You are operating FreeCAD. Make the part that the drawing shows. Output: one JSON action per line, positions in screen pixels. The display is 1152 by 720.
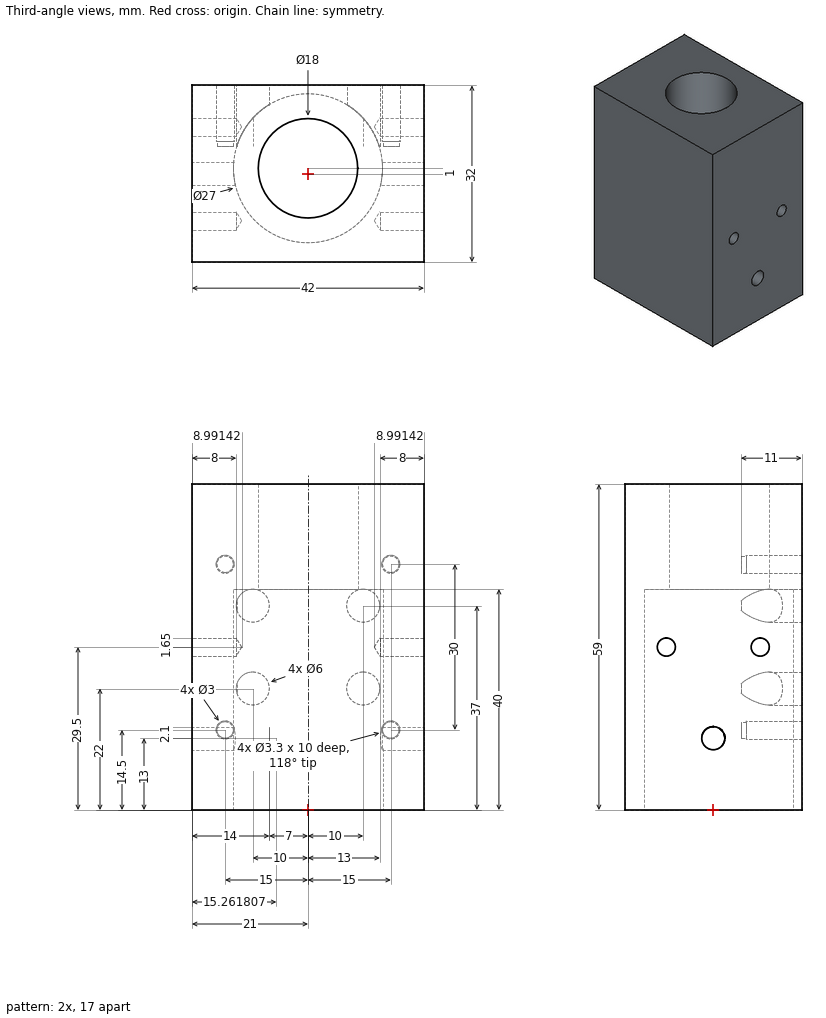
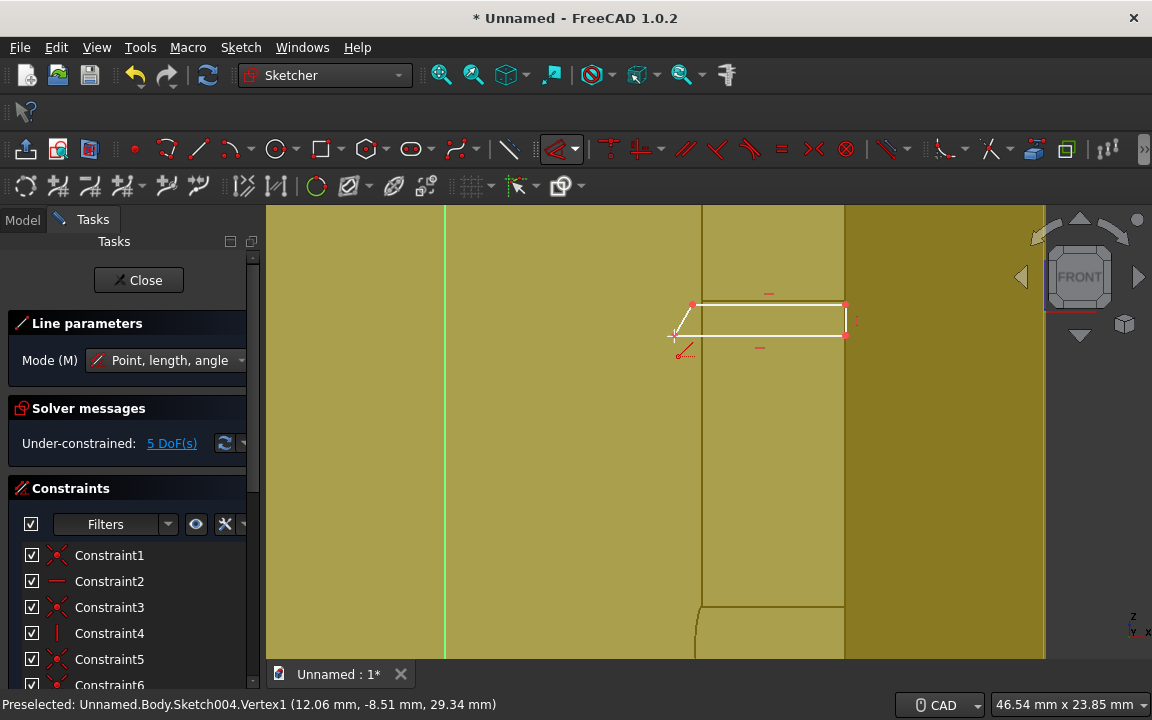
{"action": "left_click", "coordinate": [862, 333]}
{"action": "left_click", "coordinate": [913, 333]}
{"action": "key", "text": "Escape"}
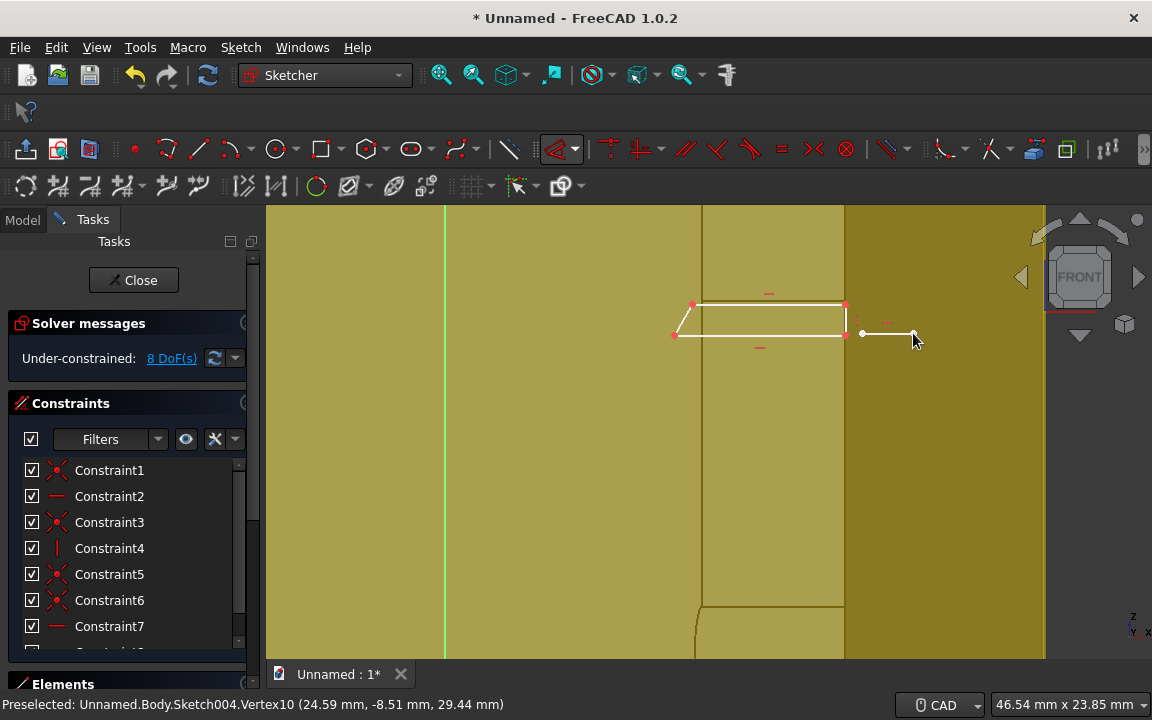
{"action": "left_click", "coordinate": [877, 334]}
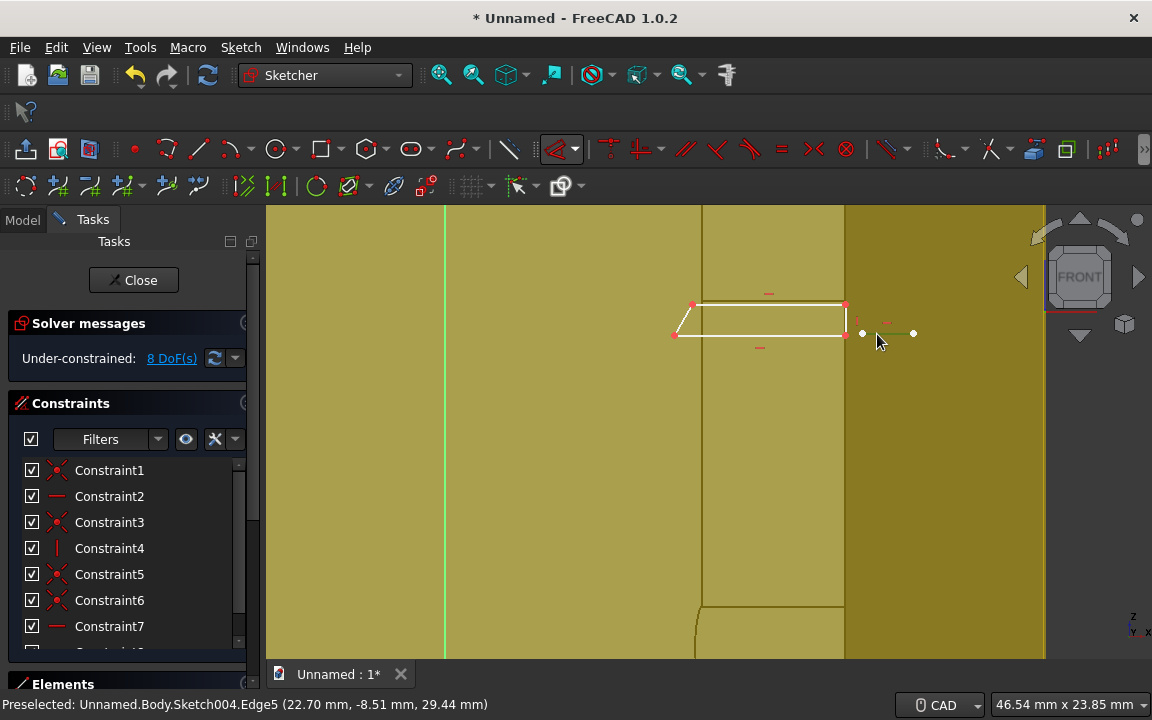
{"action": "left_click", "coordinate": [510, 150]}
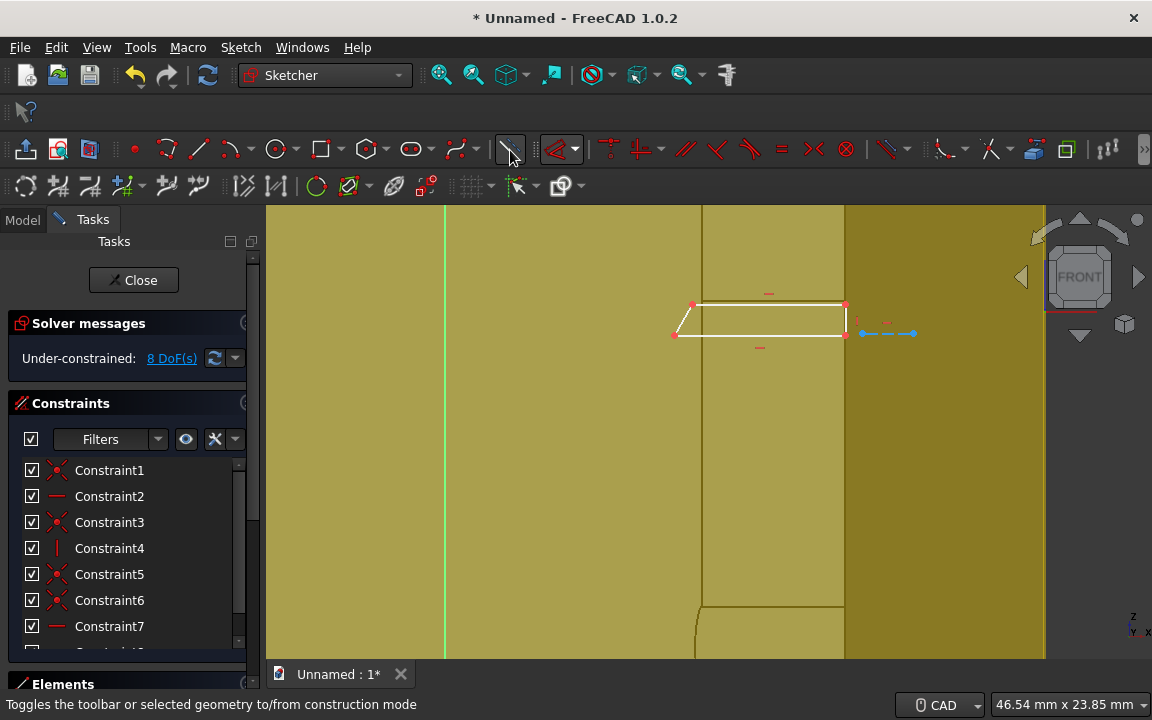
{"action": "left_click", "coordinate": [738, 305]}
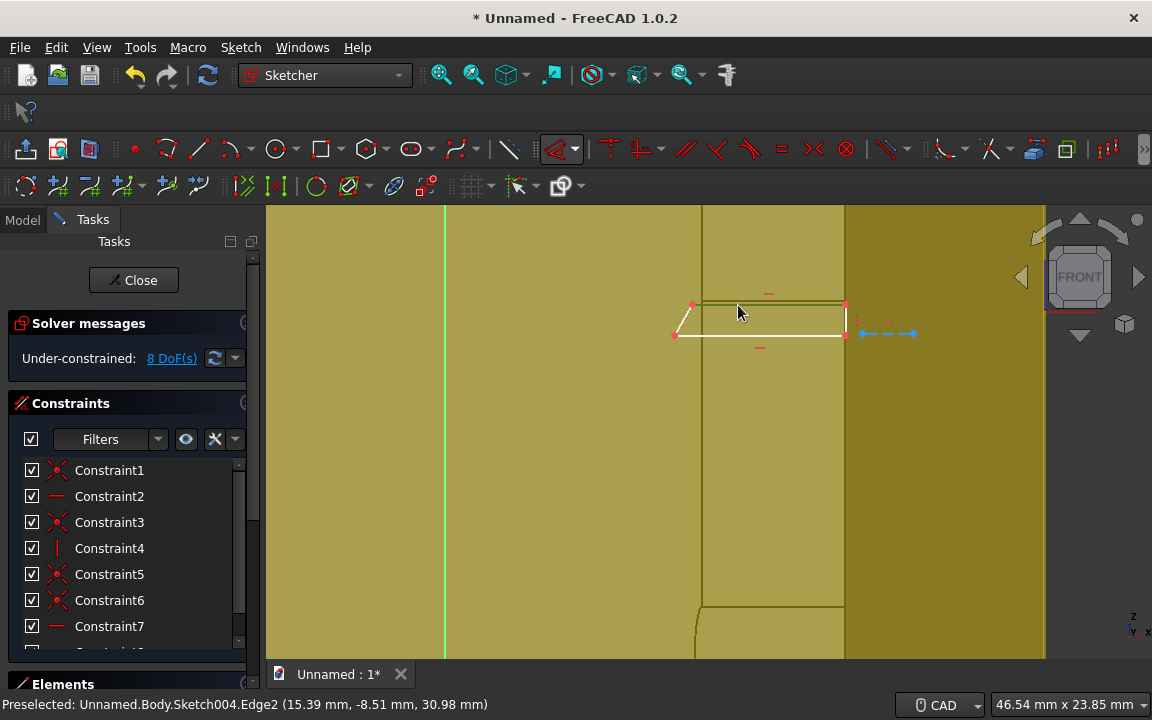
{"action": "left_click", "coordinate": [578, 150]}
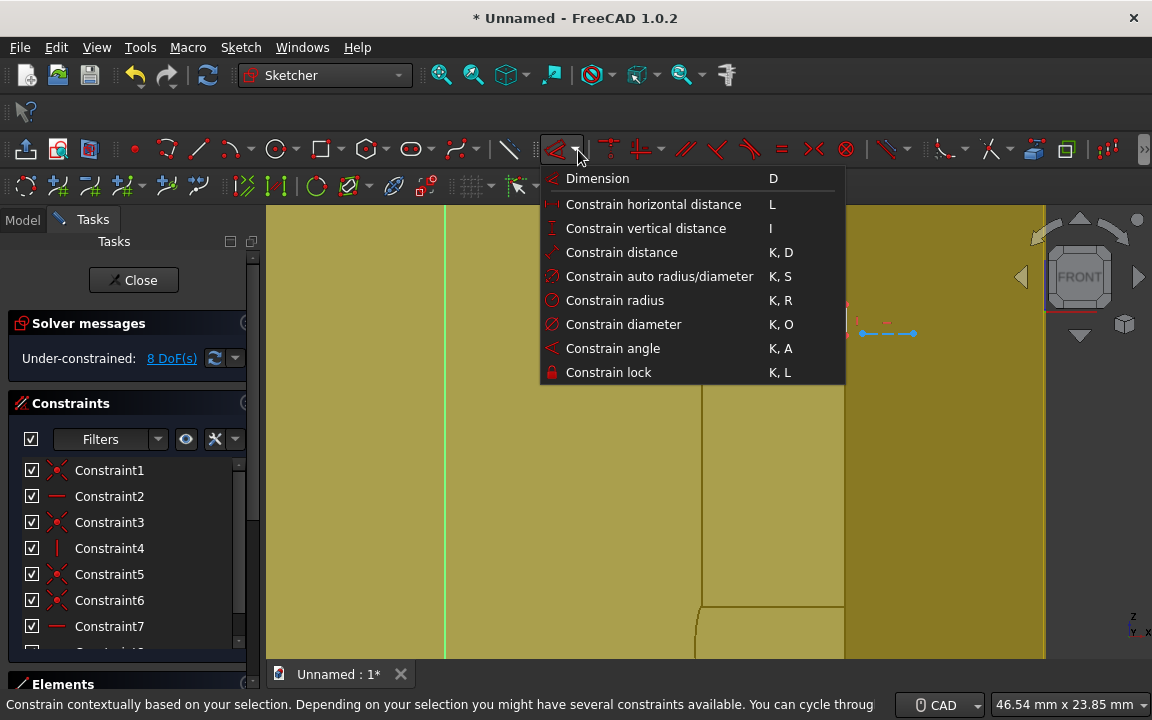
{"action": "left_click", "coordinate": [693, 204]}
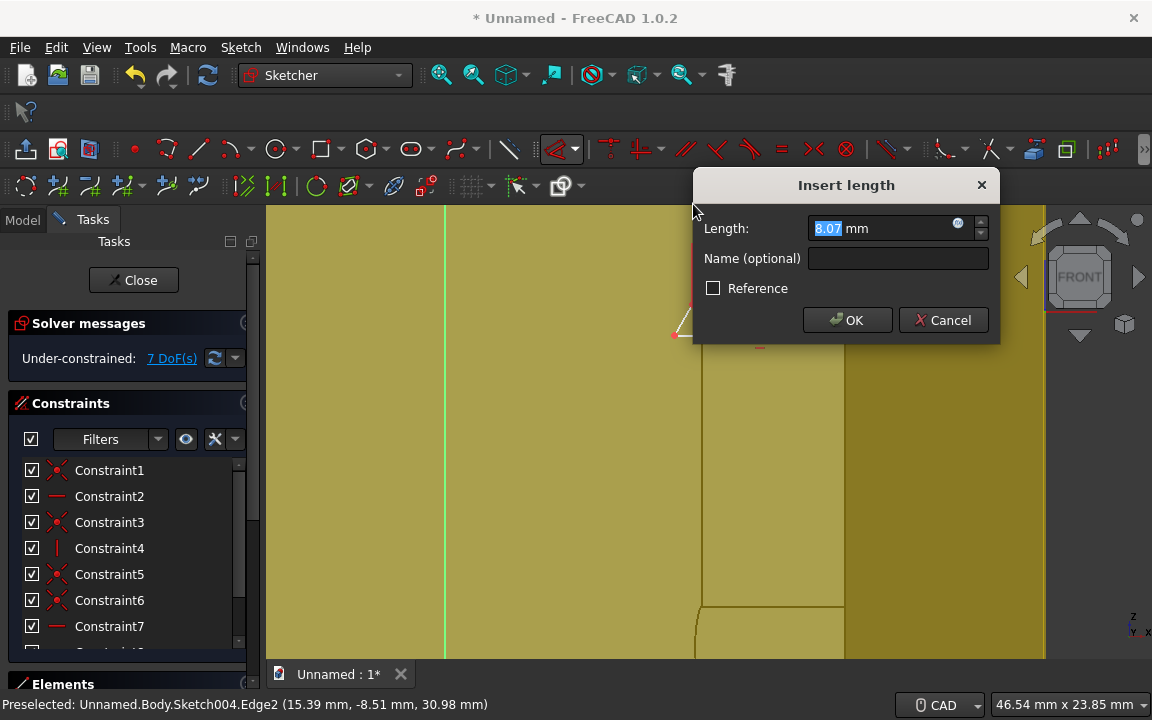
{"action": "type", "text": "8"}
{"action": "key", "text": "Return"}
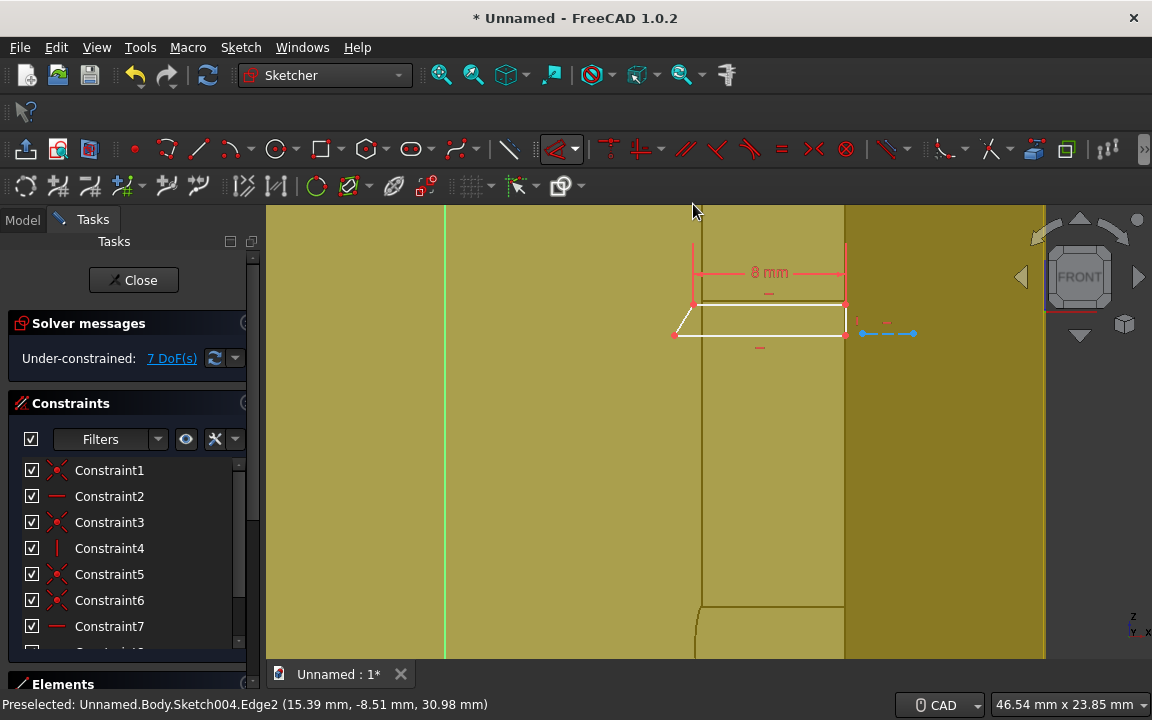
{"action": "left_click", "coordinate": [694, 305]}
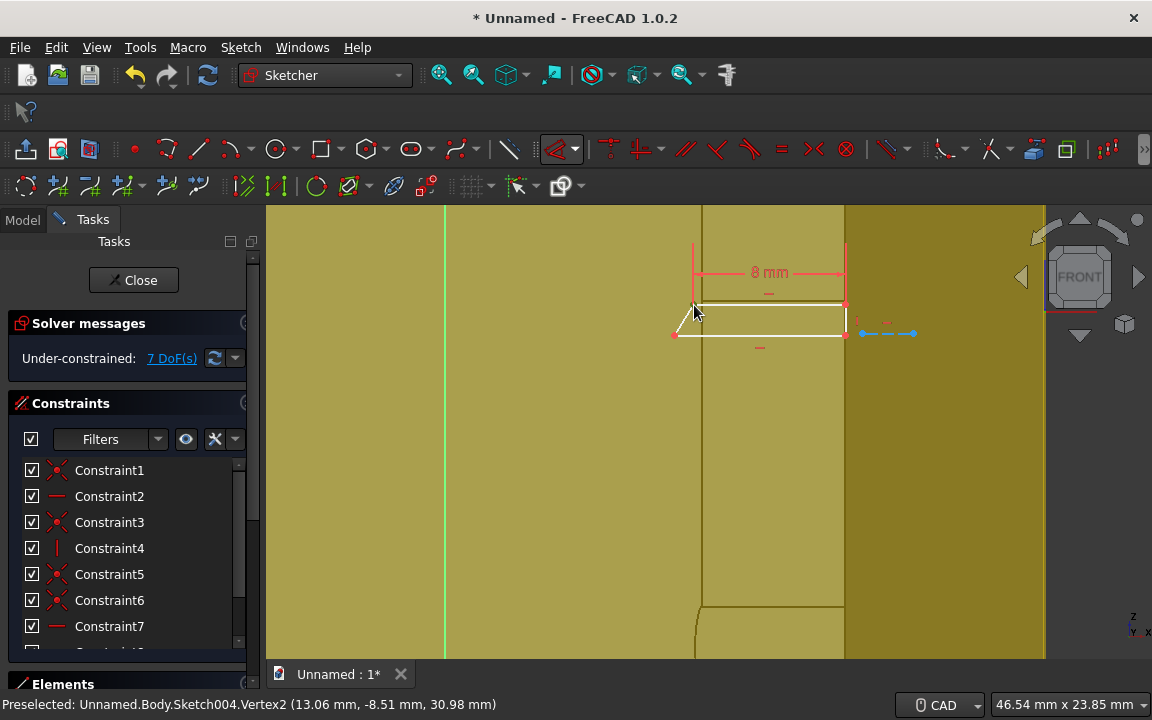
{"action": "key", "text": "l"}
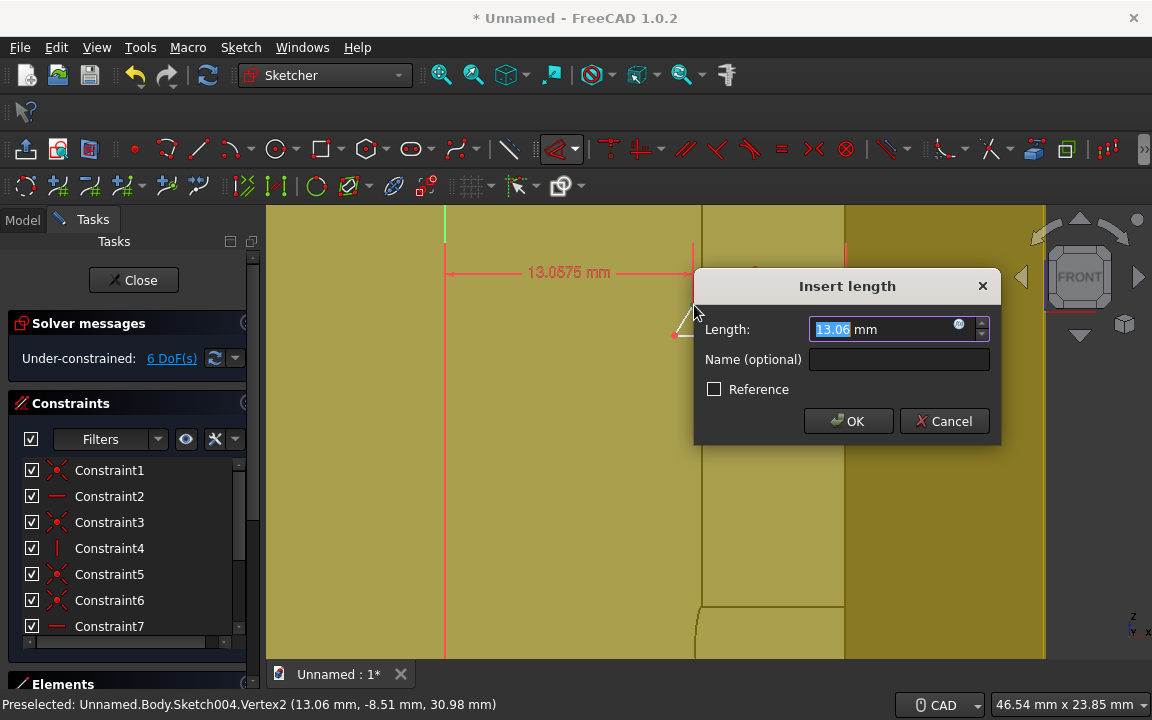
{"action": "type", "text": "13"}
{"action": "key", "text": "Return"}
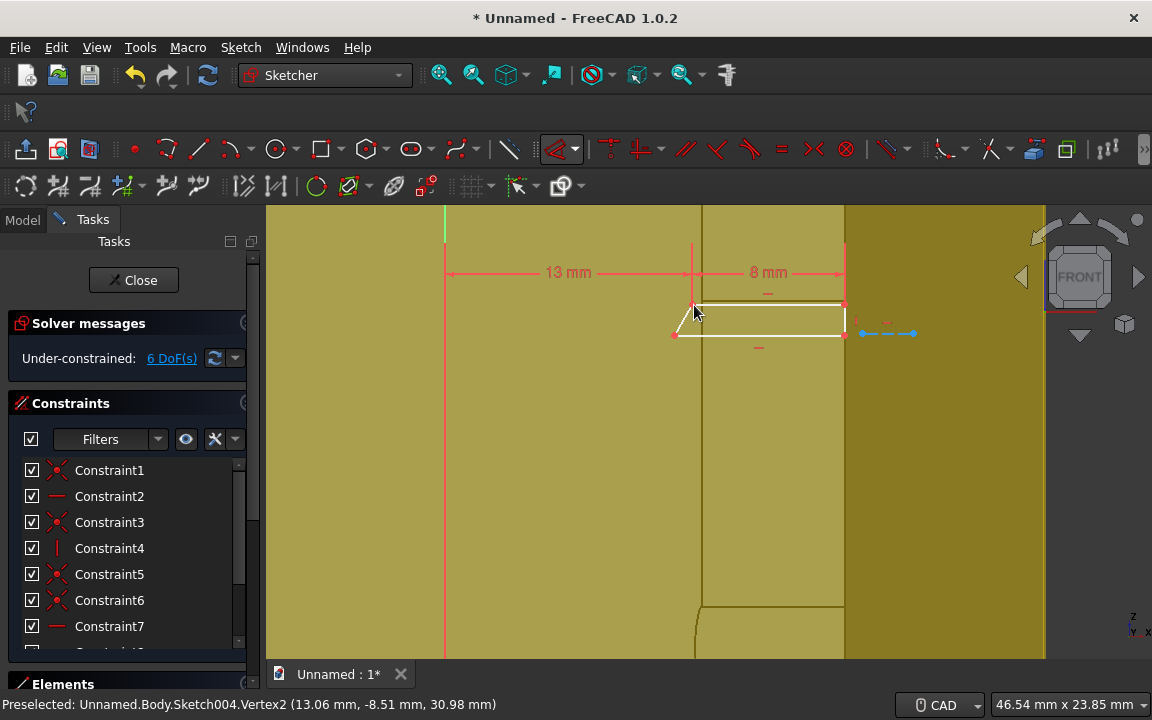
{"action": "scroll", "coordinate": [845, 314], "scroll_direction": "up", "scroll_amount": 2}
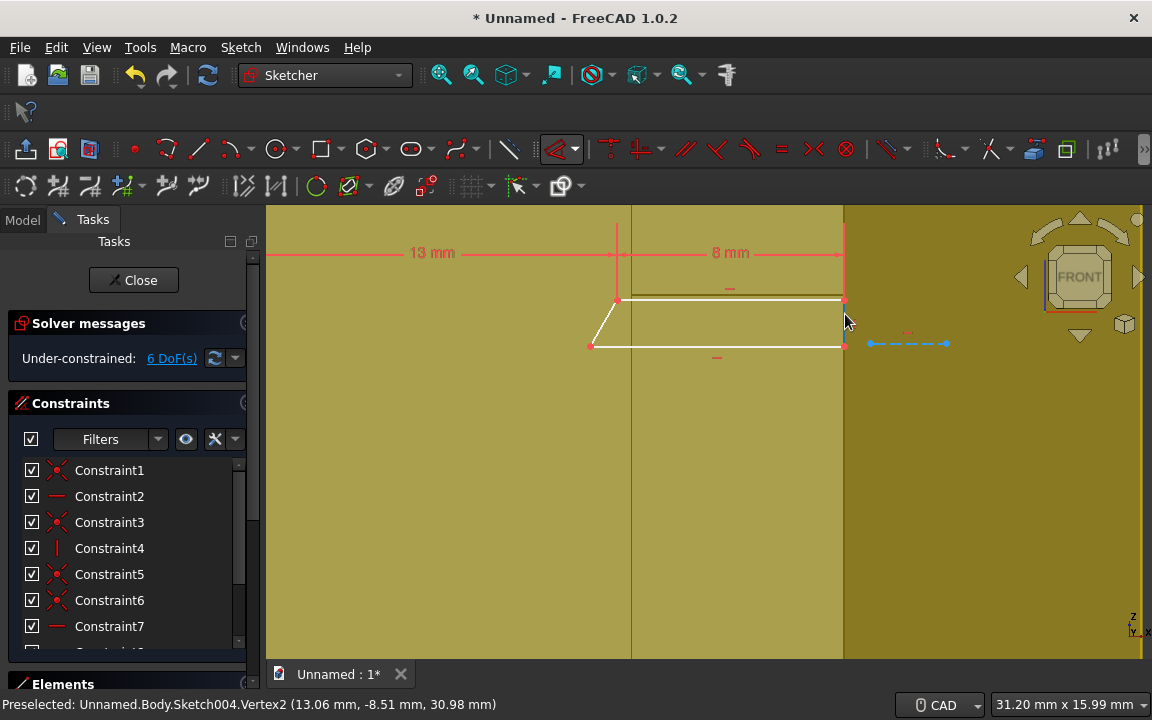
{"action": "left_click", "coordinate": [844, 314]}